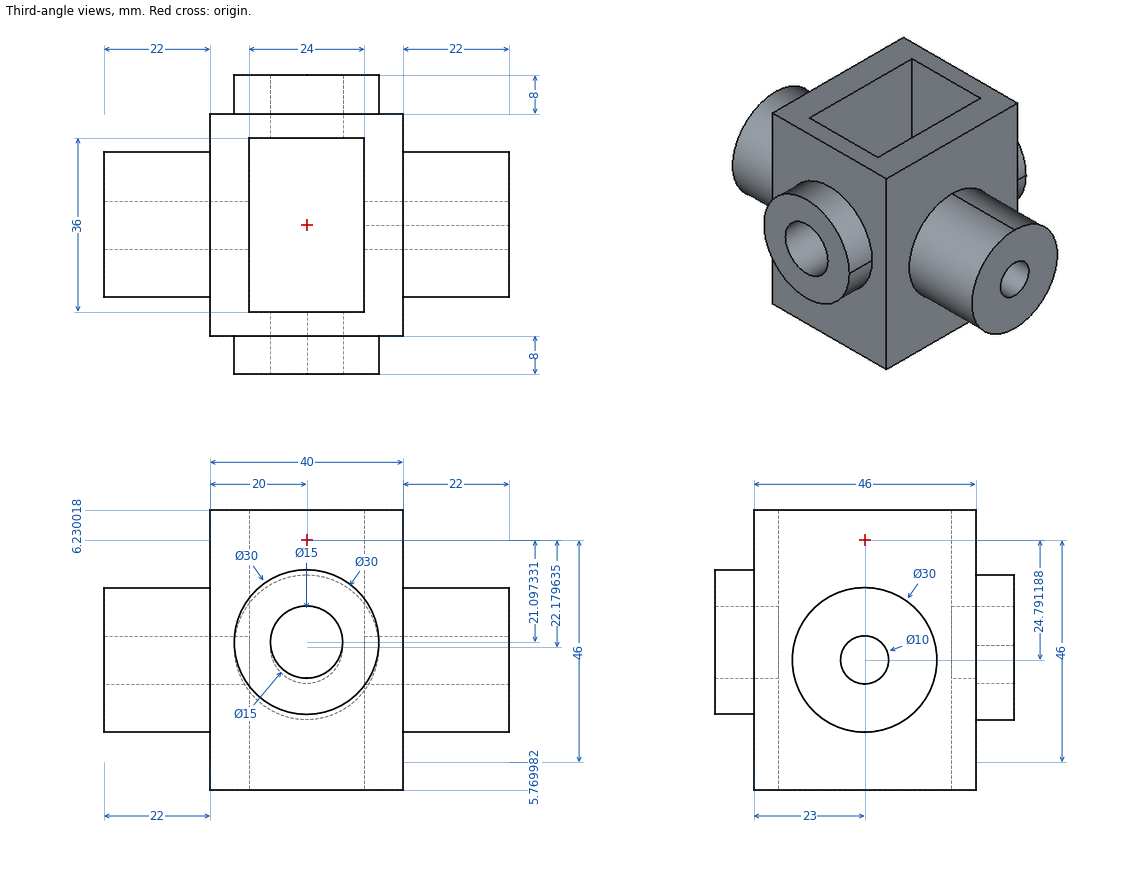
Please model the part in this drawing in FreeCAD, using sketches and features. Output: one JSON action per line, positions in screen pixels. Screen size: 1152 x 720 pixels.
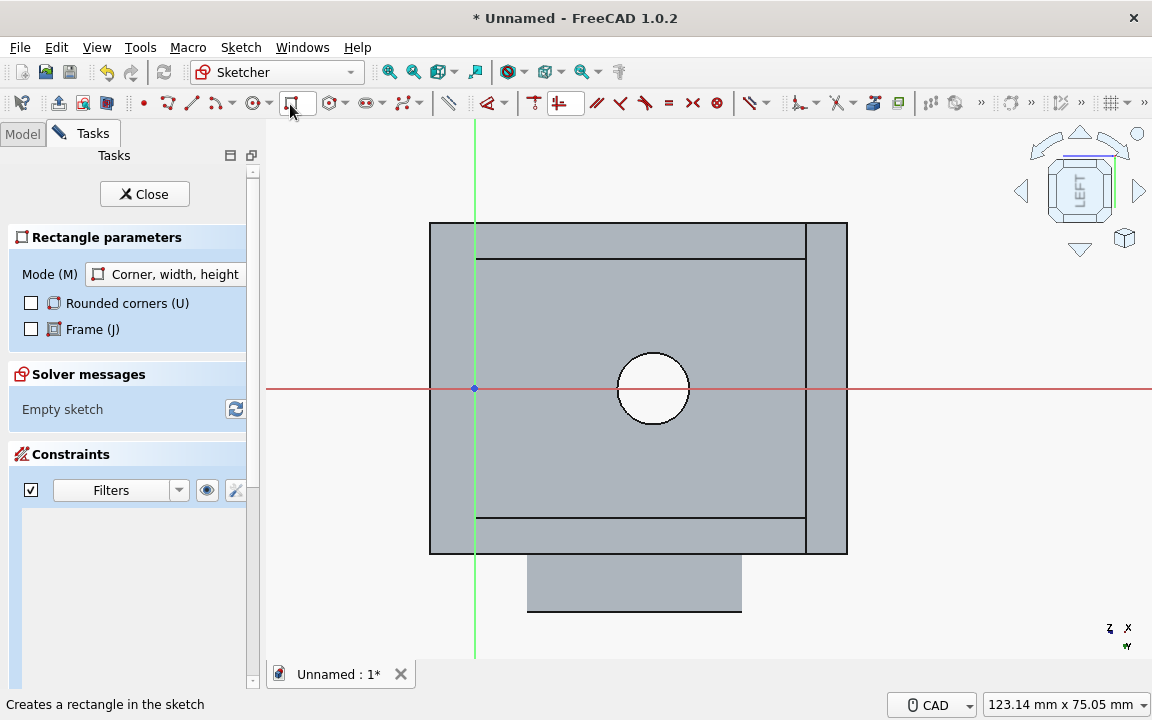
{"action": "left_click", "coordinate": [475, 223]}
{"action": "left_click", "coordinate": [806, 554]}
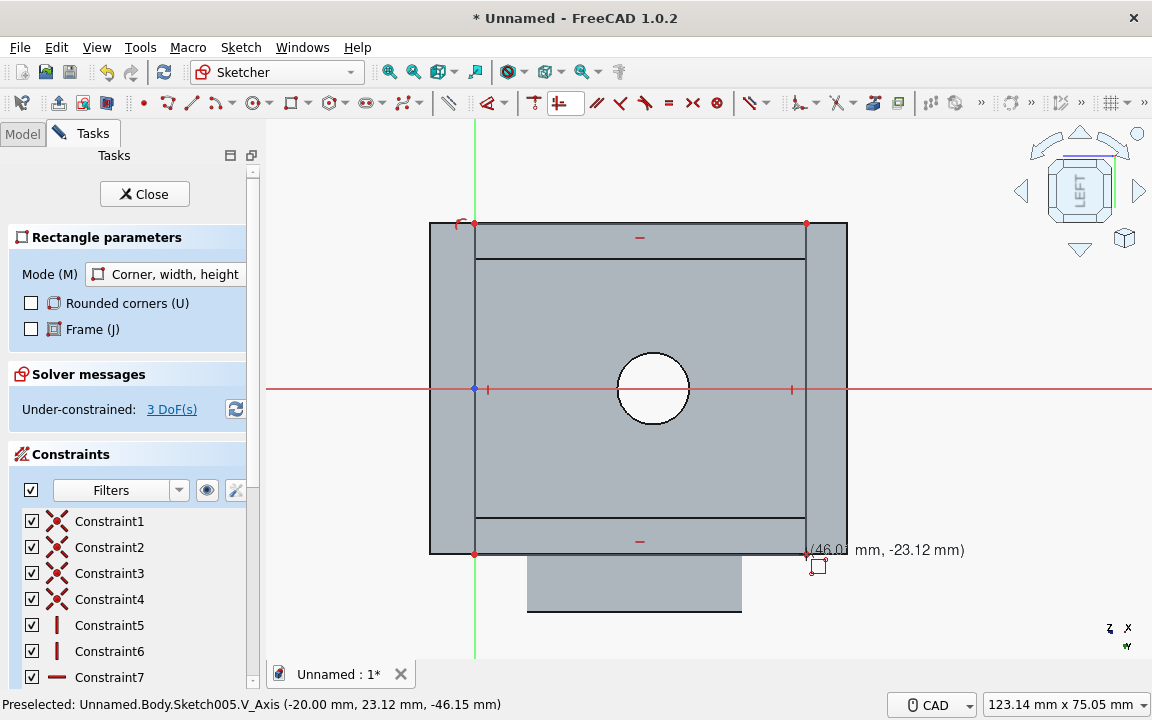
{"action": "left_click", "coordinate": [254, 104]}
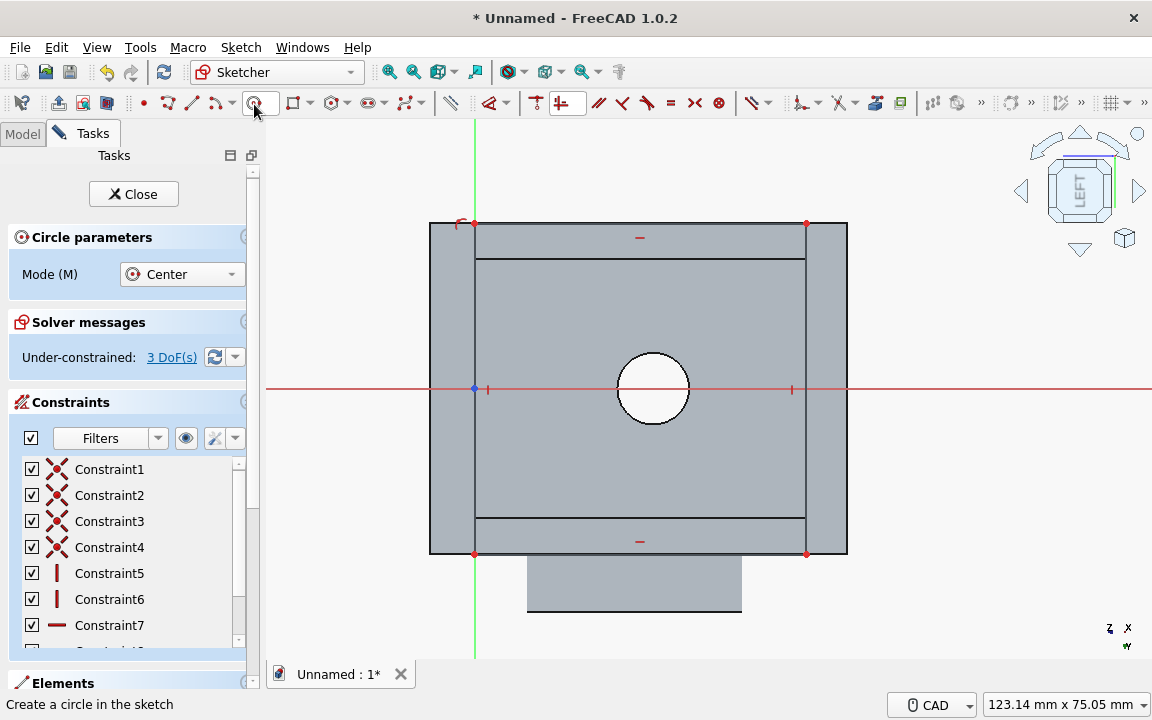
{"action": "left_click", "coordinate": [653, 389]}
{"action": "left_click", "coordinate": [730, 312]}
{"action": "key", "text": "Escape"}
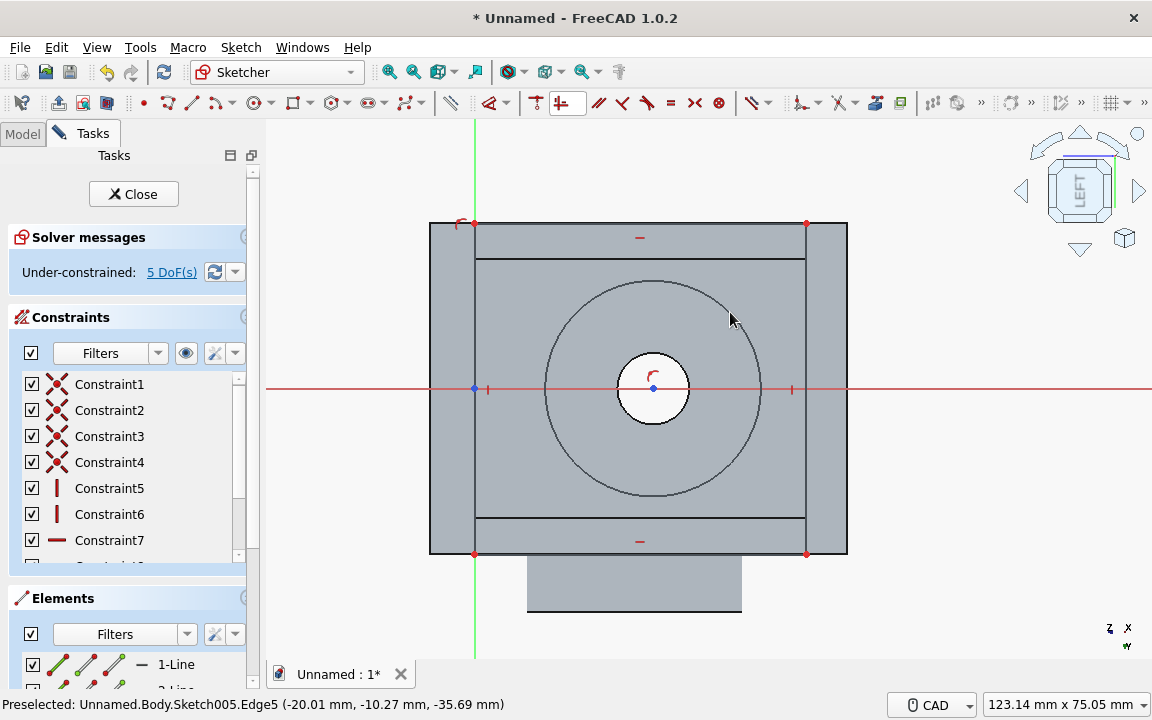
{"action": "left_click", "coordinate": [490, 104]}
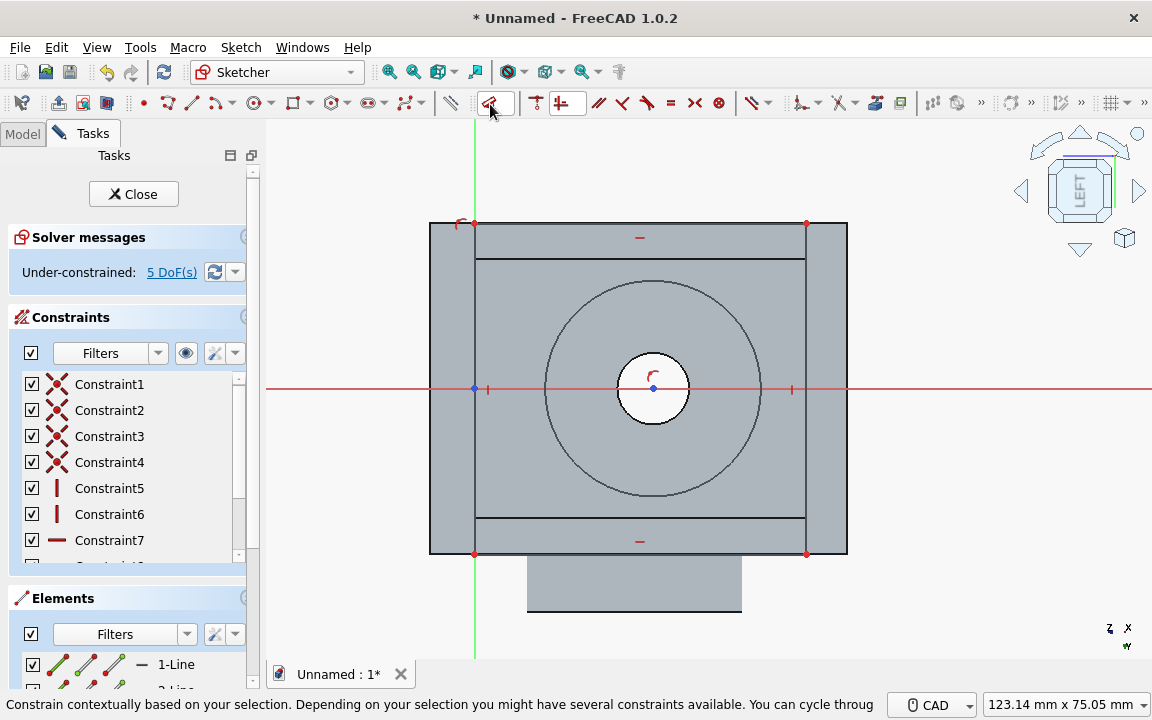
{"action": "left_click", "coordinate": [729, 312]}
{"action": "left_click", "coordinate": [752, 289]}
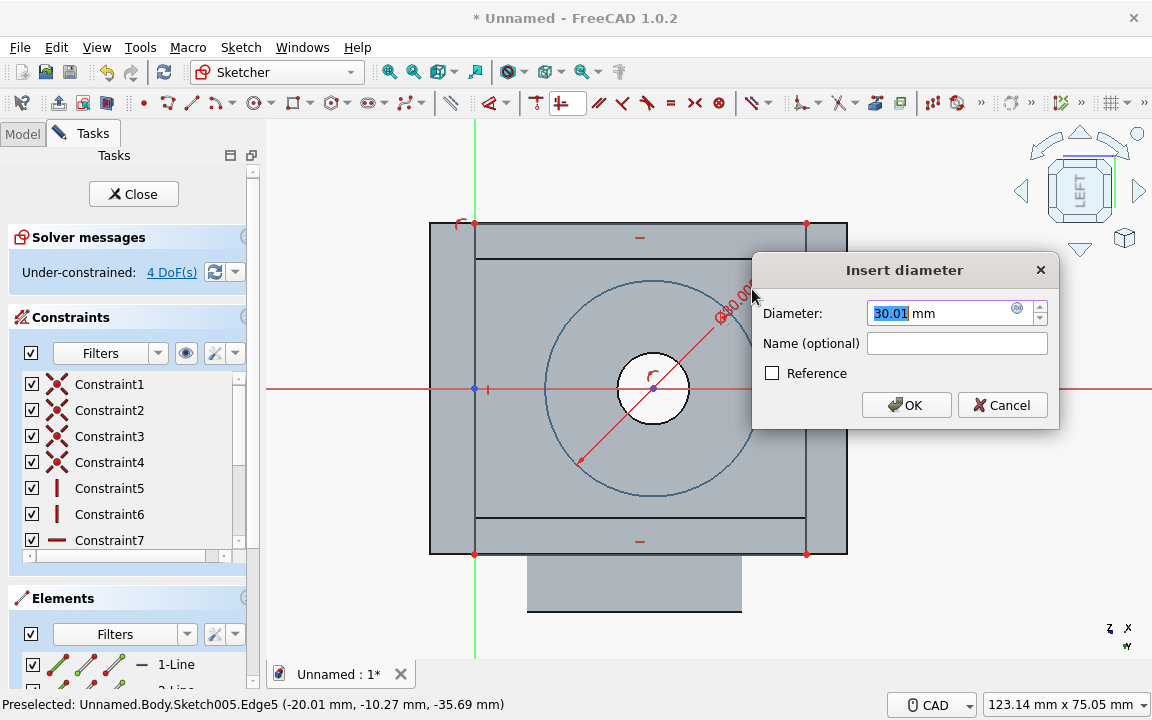
{"action": "type", "text": "30"}
{"action": "key", "text": "Return"}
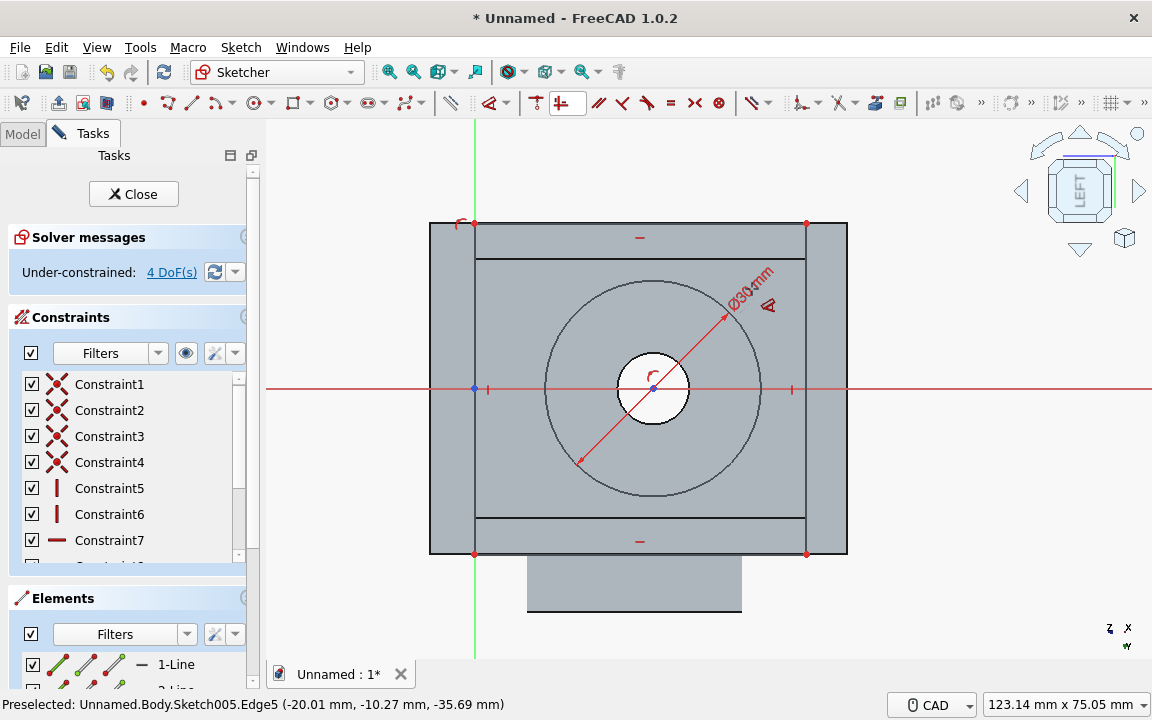
{"action": "left_click", "coordinate": [475, 323]}
{"action": "left_click", "coordinate": [441, 313]}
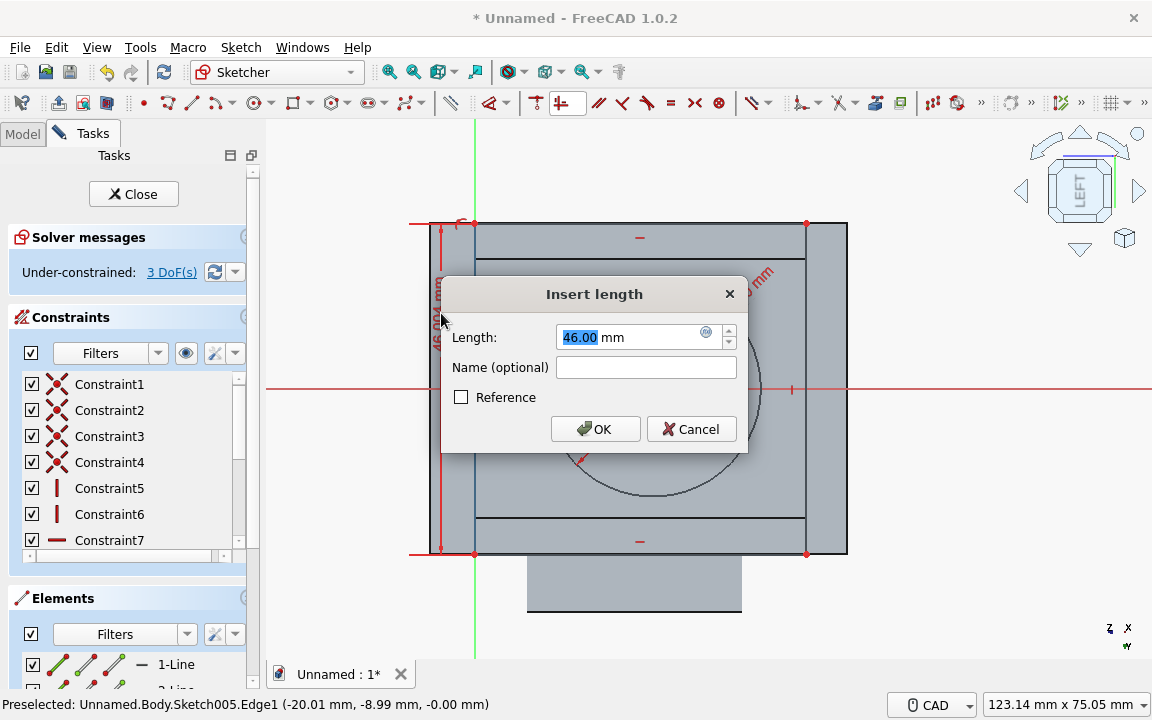
{"action": "type", "text": "46"}
{"action": "key", "text": "Return"}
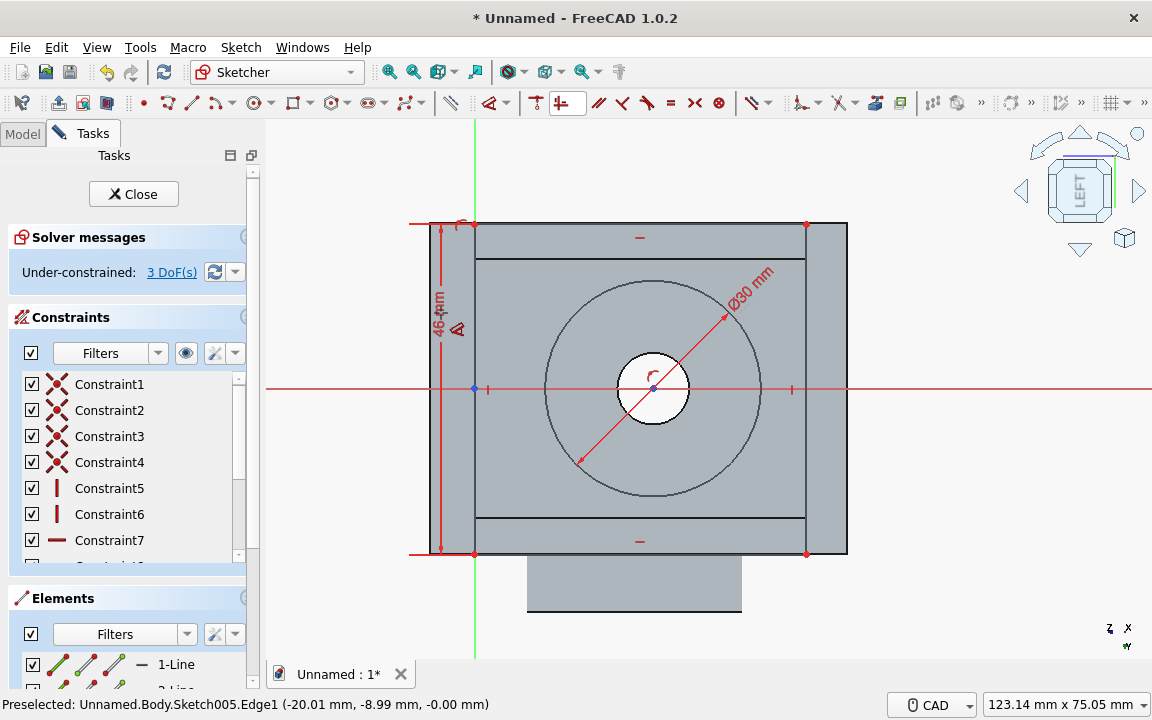
{"action": "left_click", "coordinate": [574, 555]}
{"action": "left_click", "coordinate": [640, 589]}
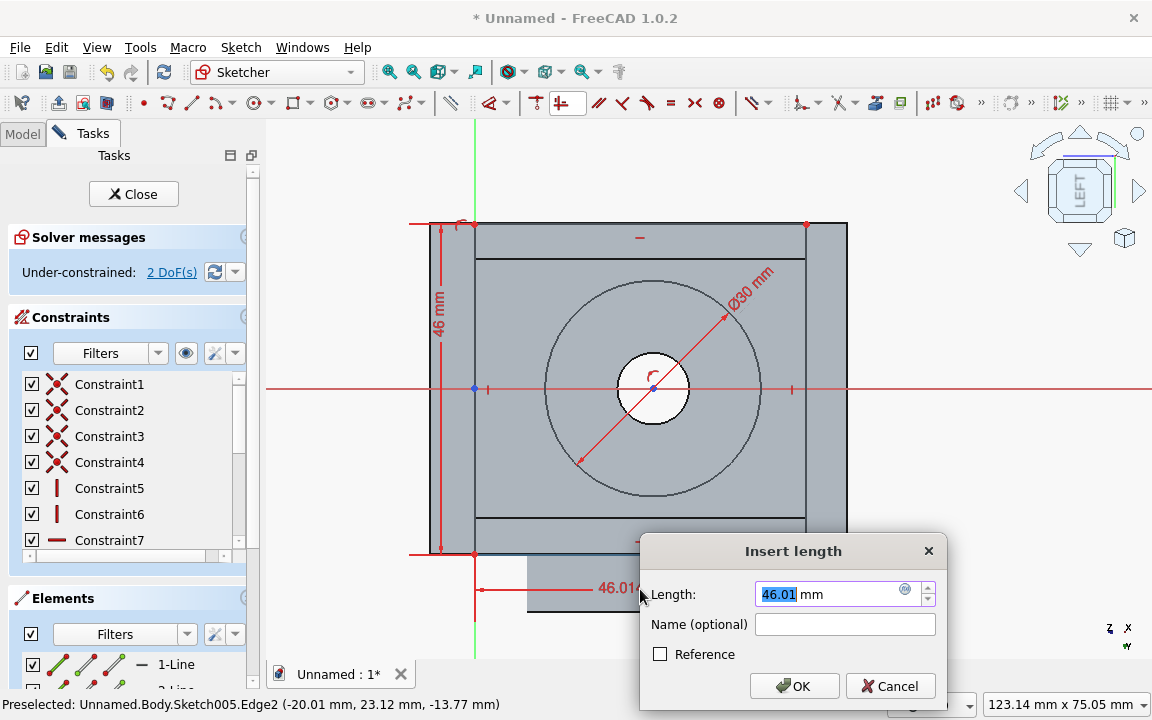
{"action": "type", "text": "46"}
{"action": "key", "text": "Return"}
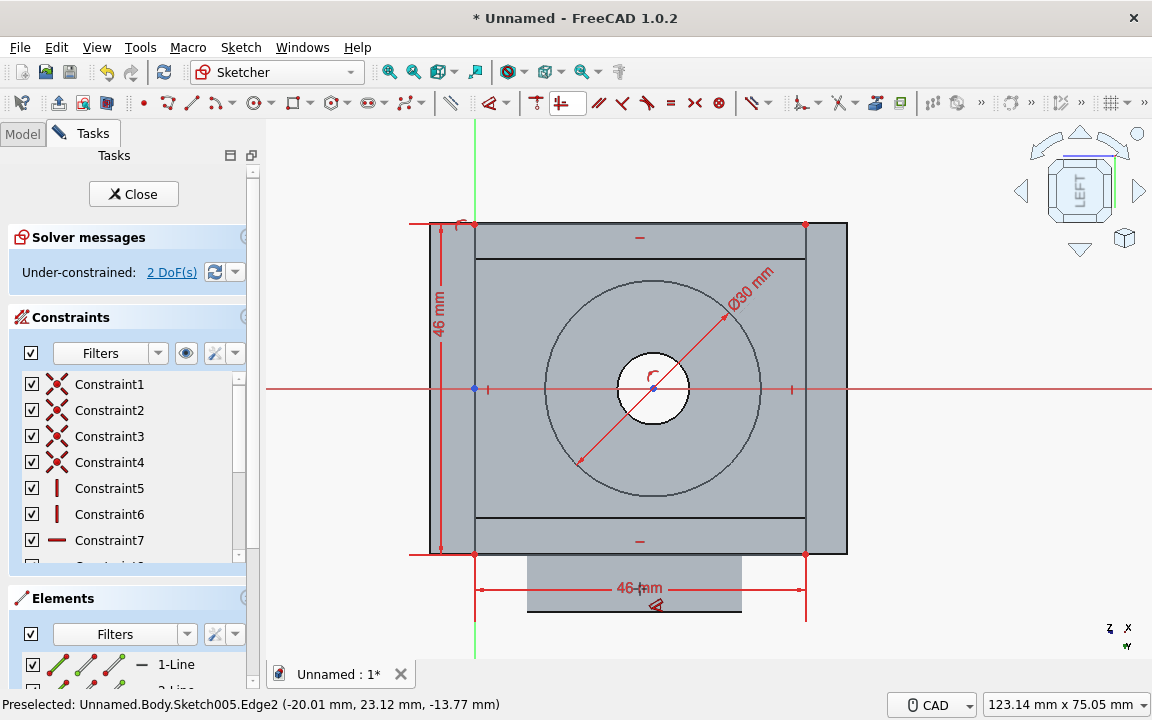
{"action": "left_click", "coordinate": [475, 224]}
{"action": "left_click", "coordinate": [441, 268]}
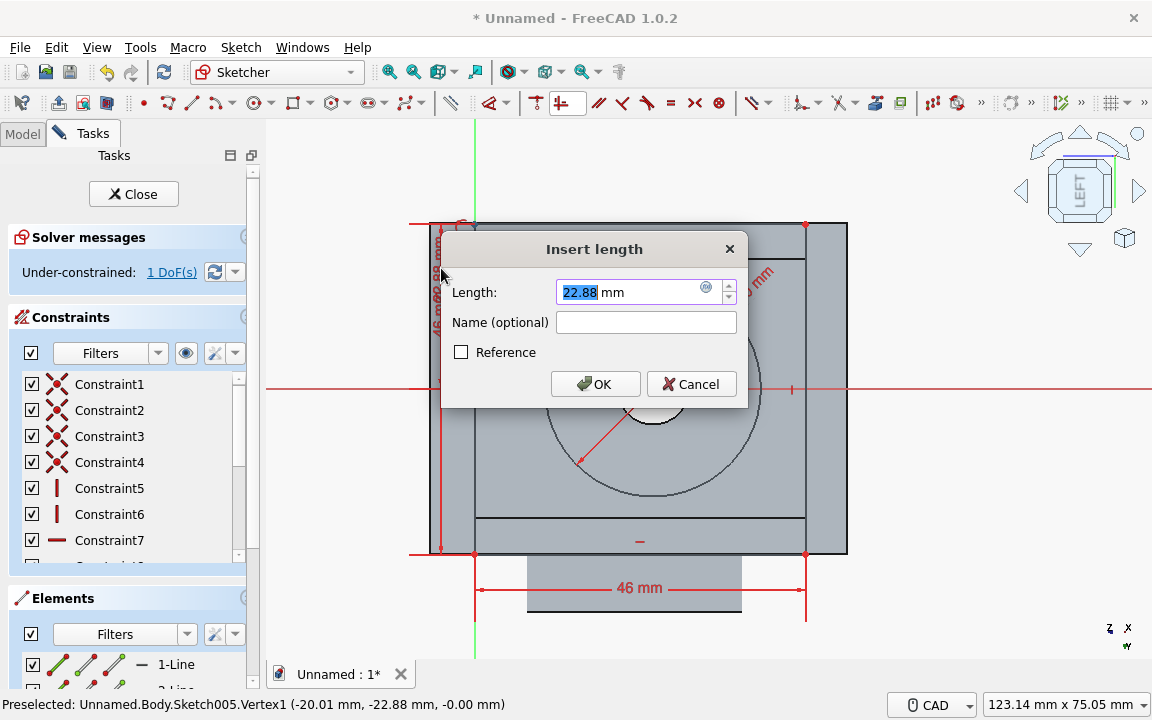
{"action": "type", "text": "23"}
{"action": "key", "text": "Return"}